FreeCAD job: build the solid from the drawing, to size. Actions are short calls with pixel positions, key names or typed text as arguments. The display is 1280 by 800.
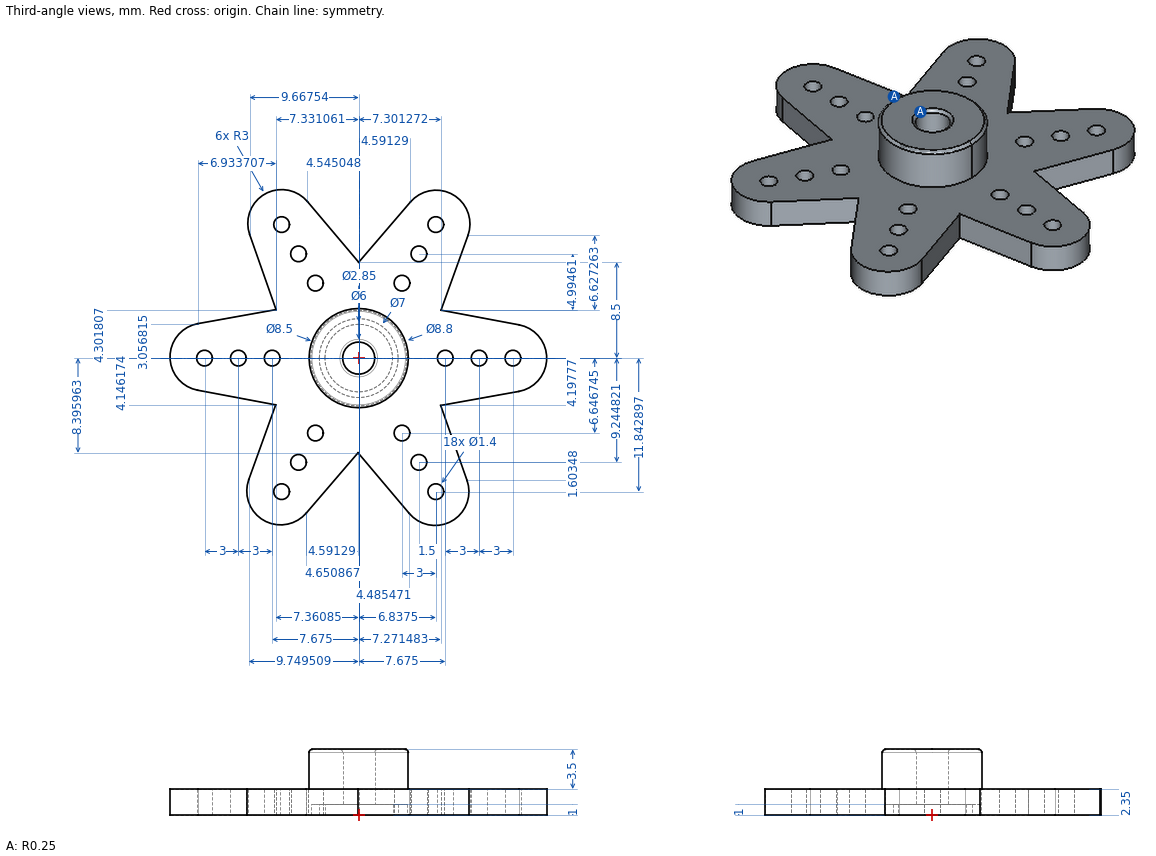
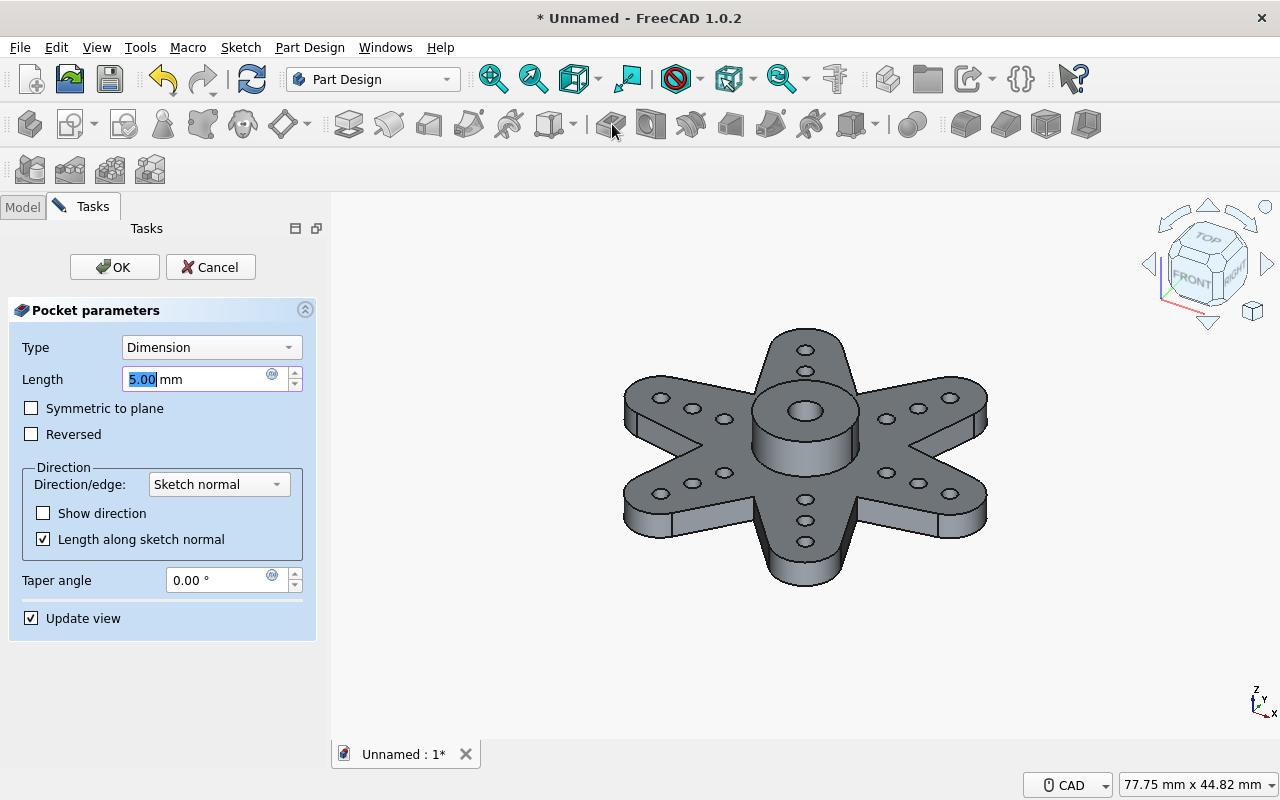
click(212, 348)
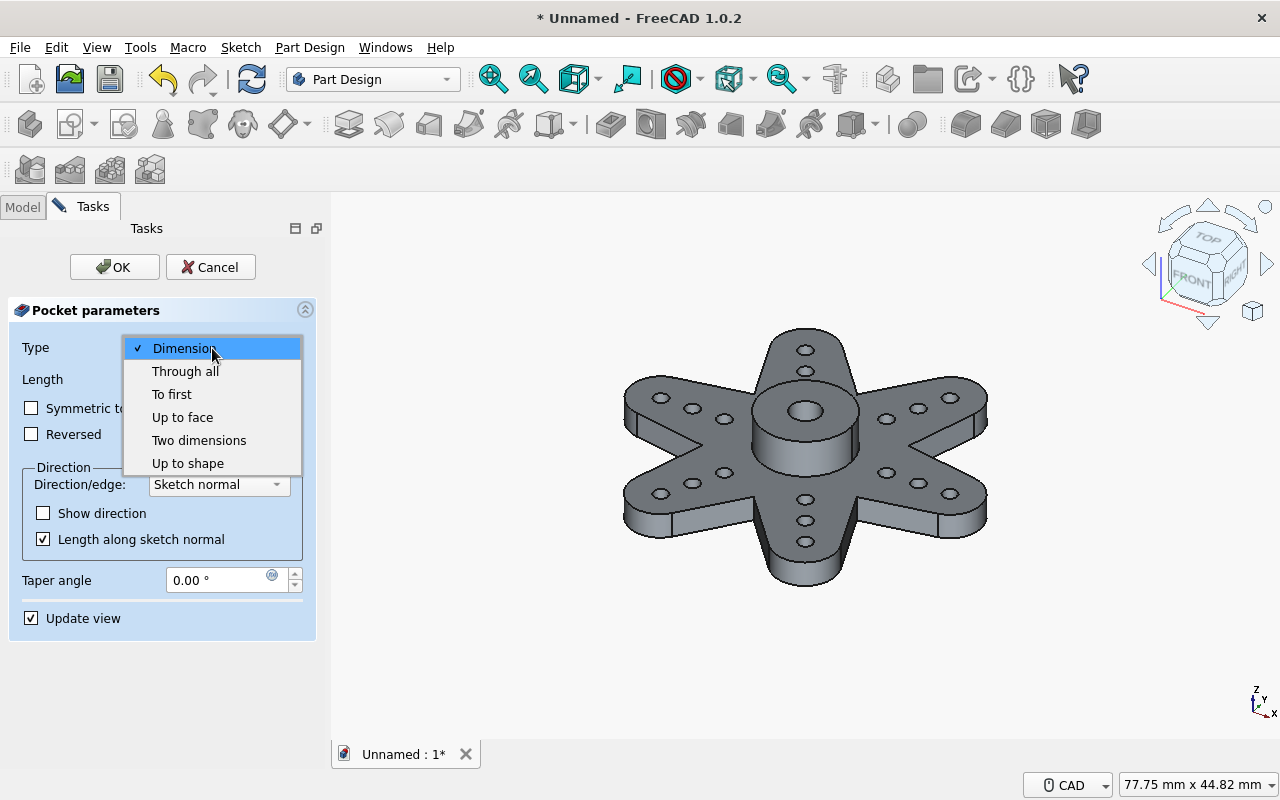
click(212, 372)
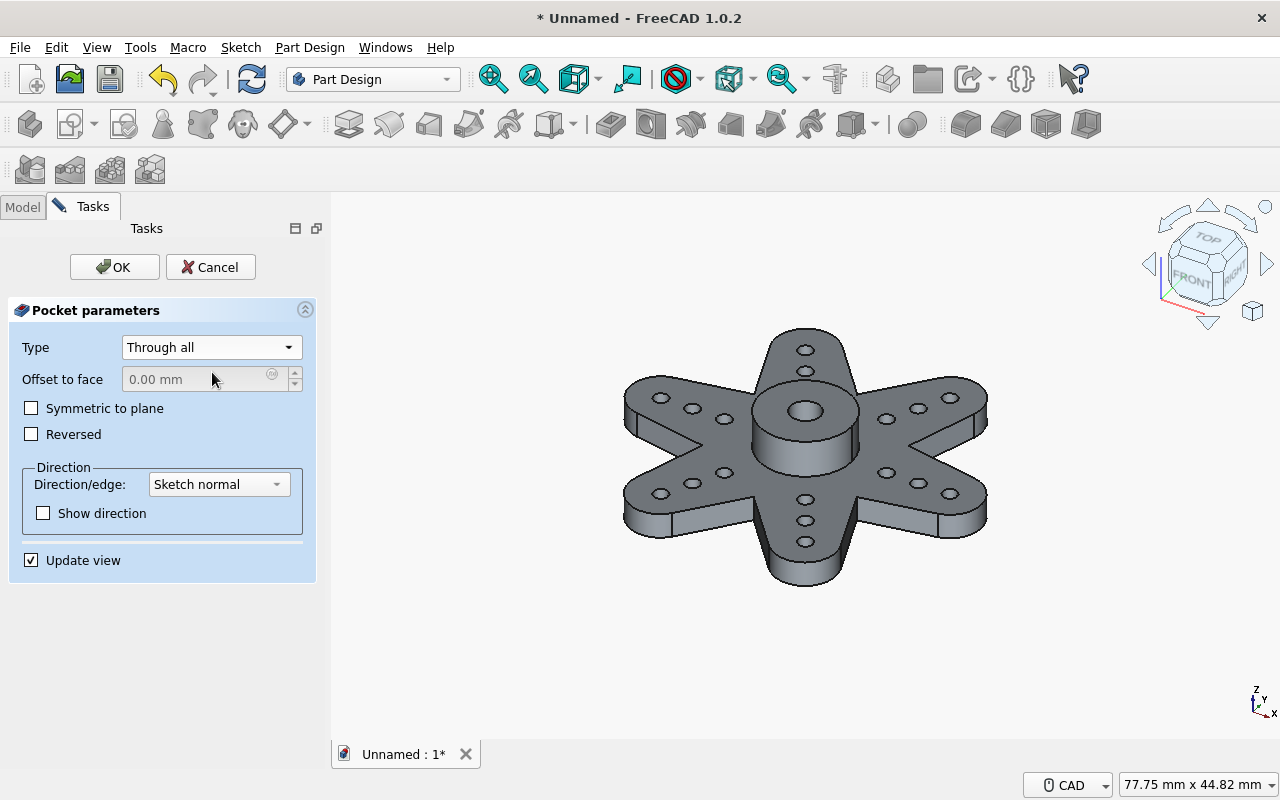
click(115, 267)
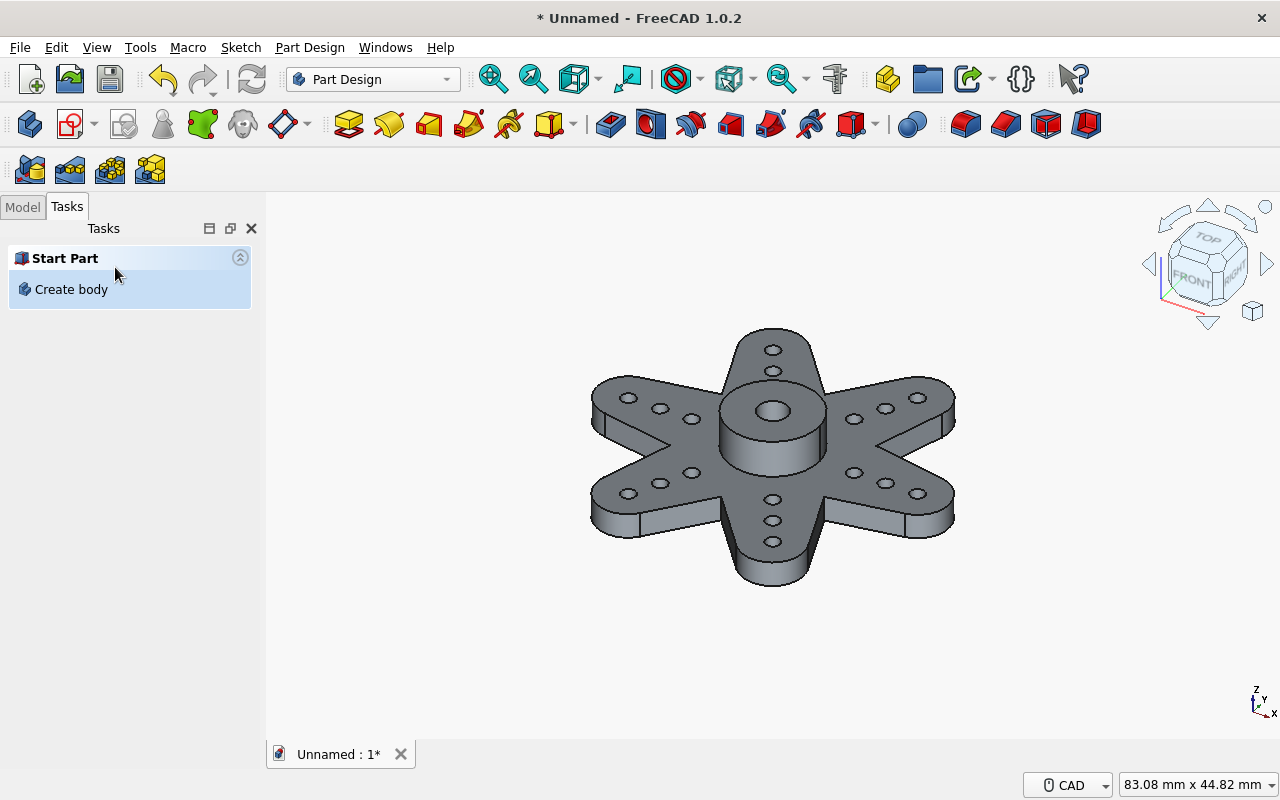
click(726, 395)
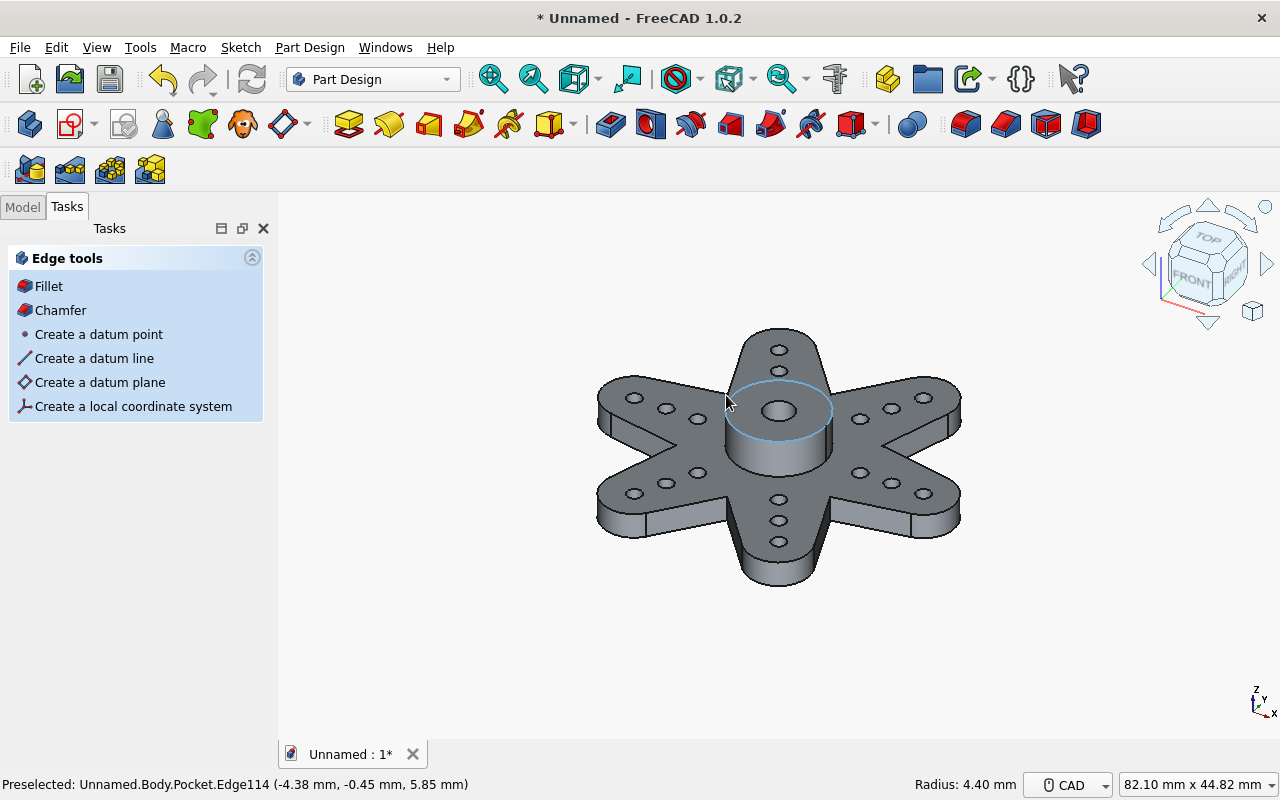
click(764, 405, ctrl)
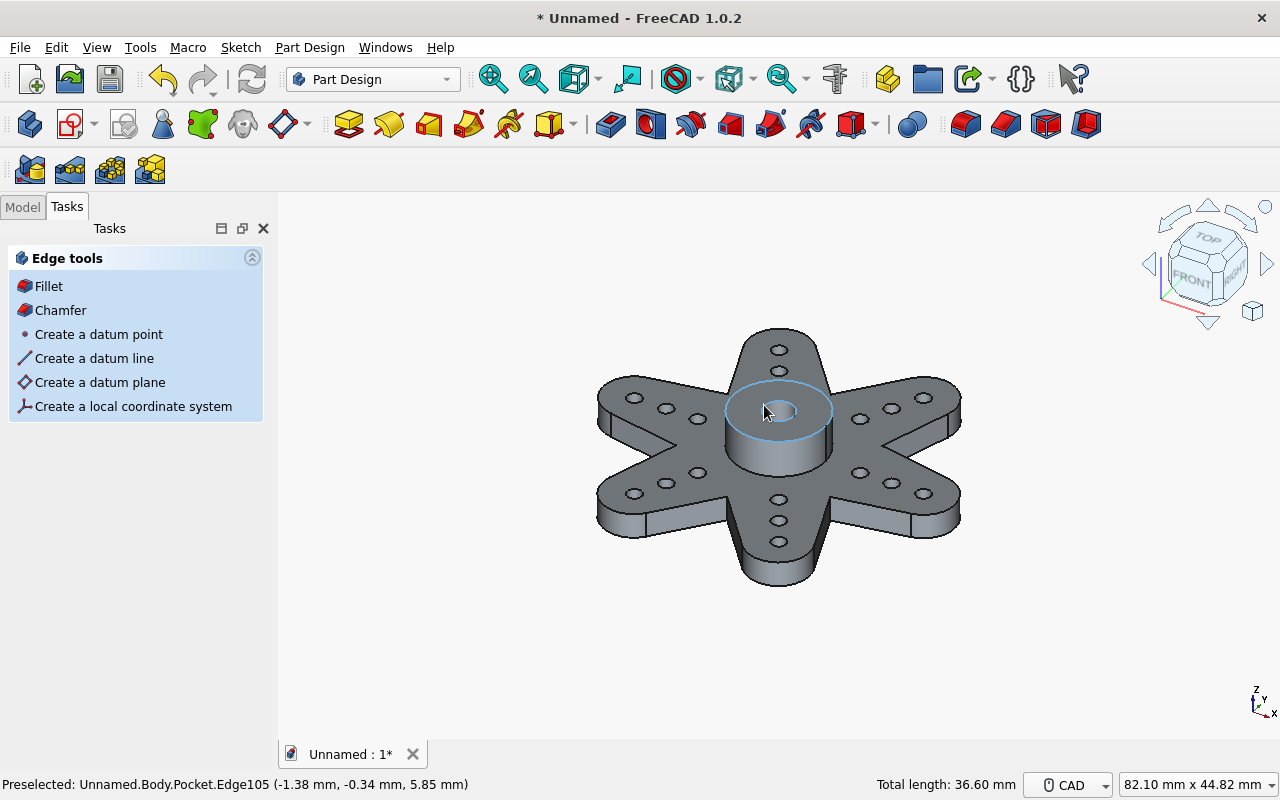
click(966, 124)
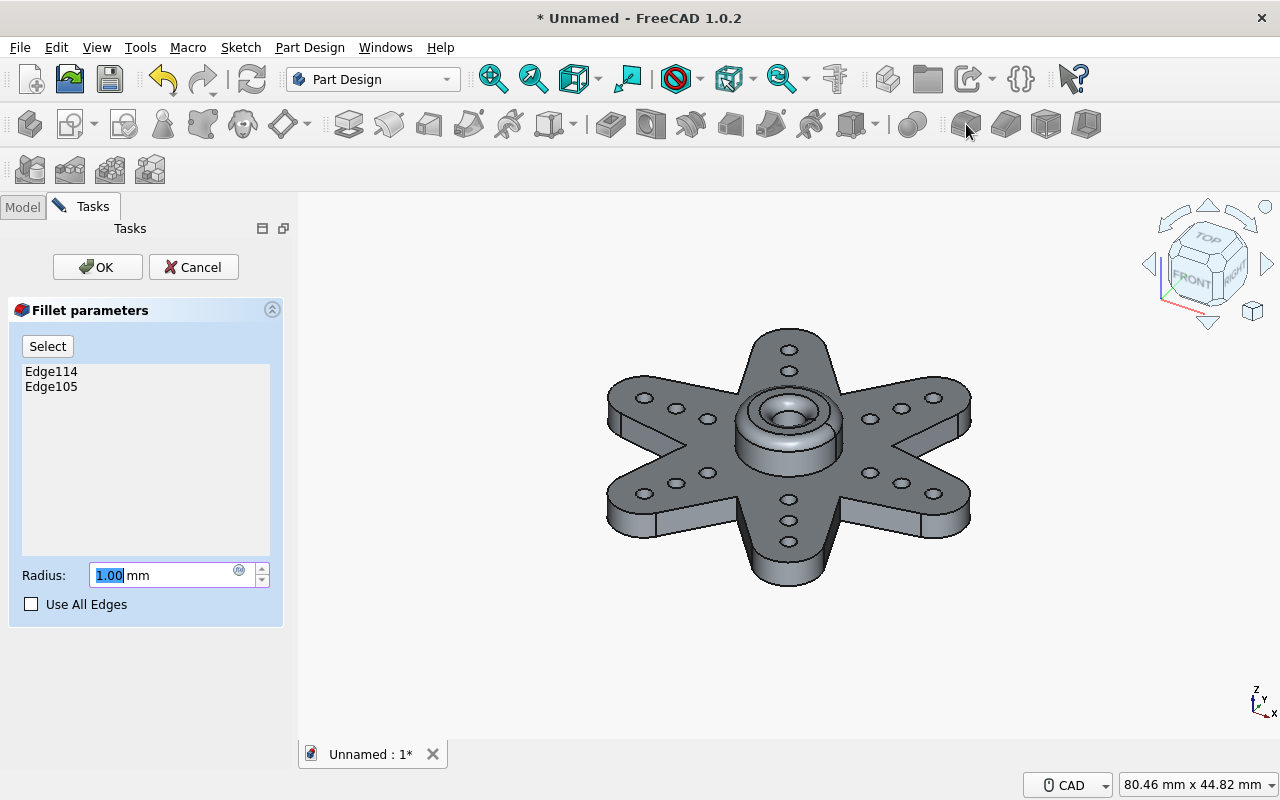
text(0.25)
key(Tab)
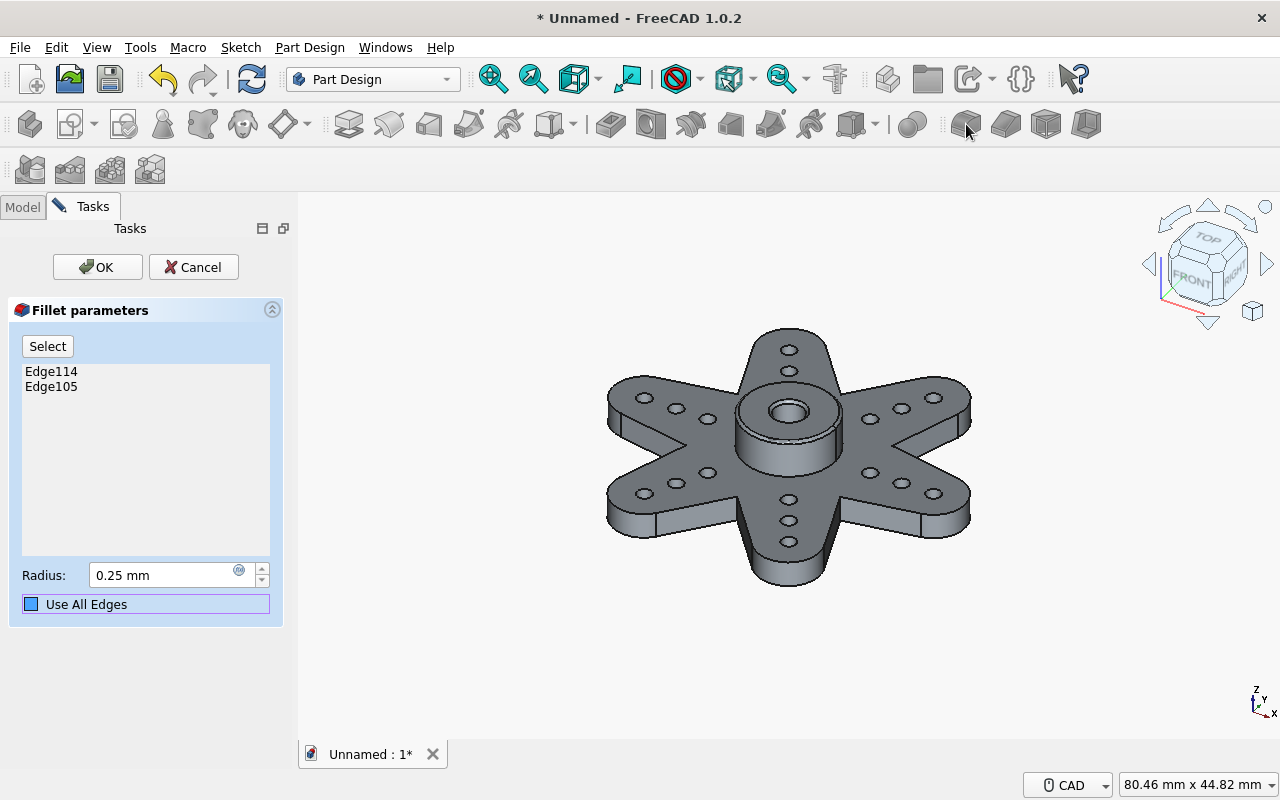
click(98, 267)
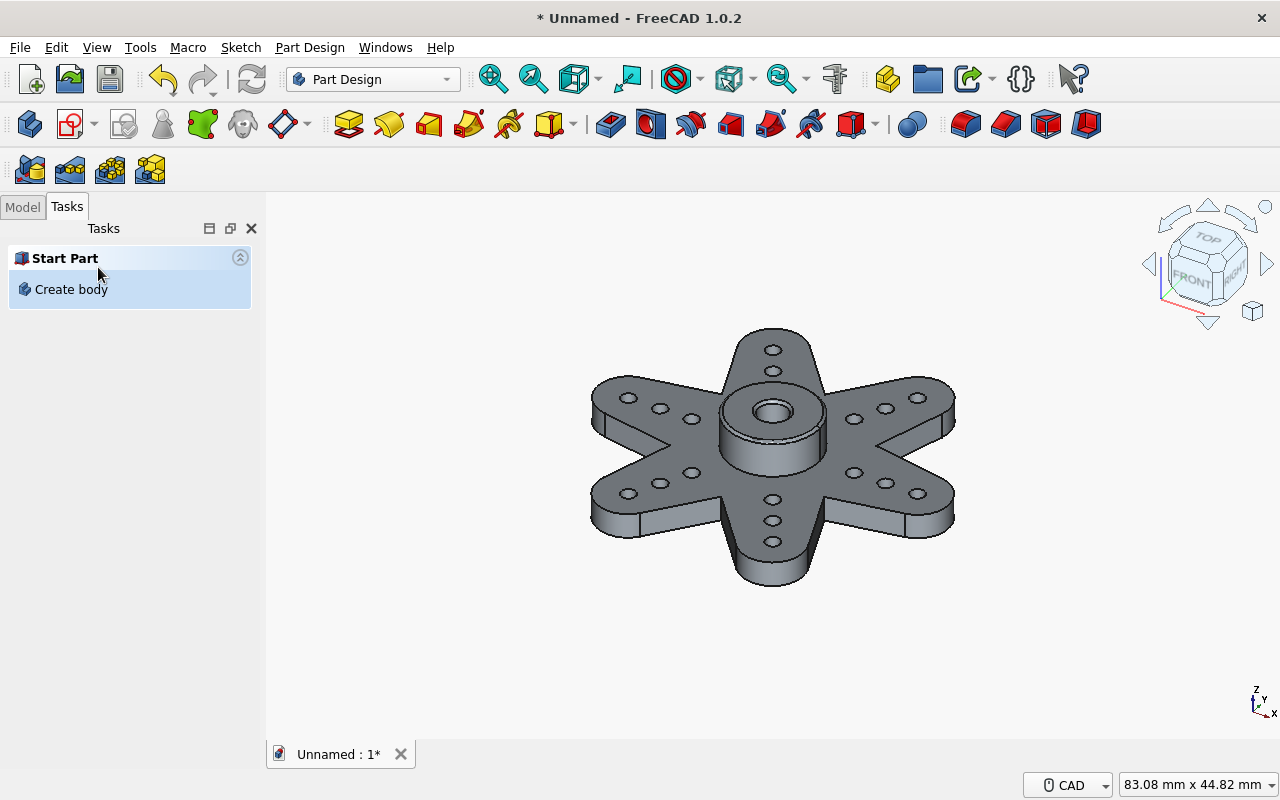
key(5)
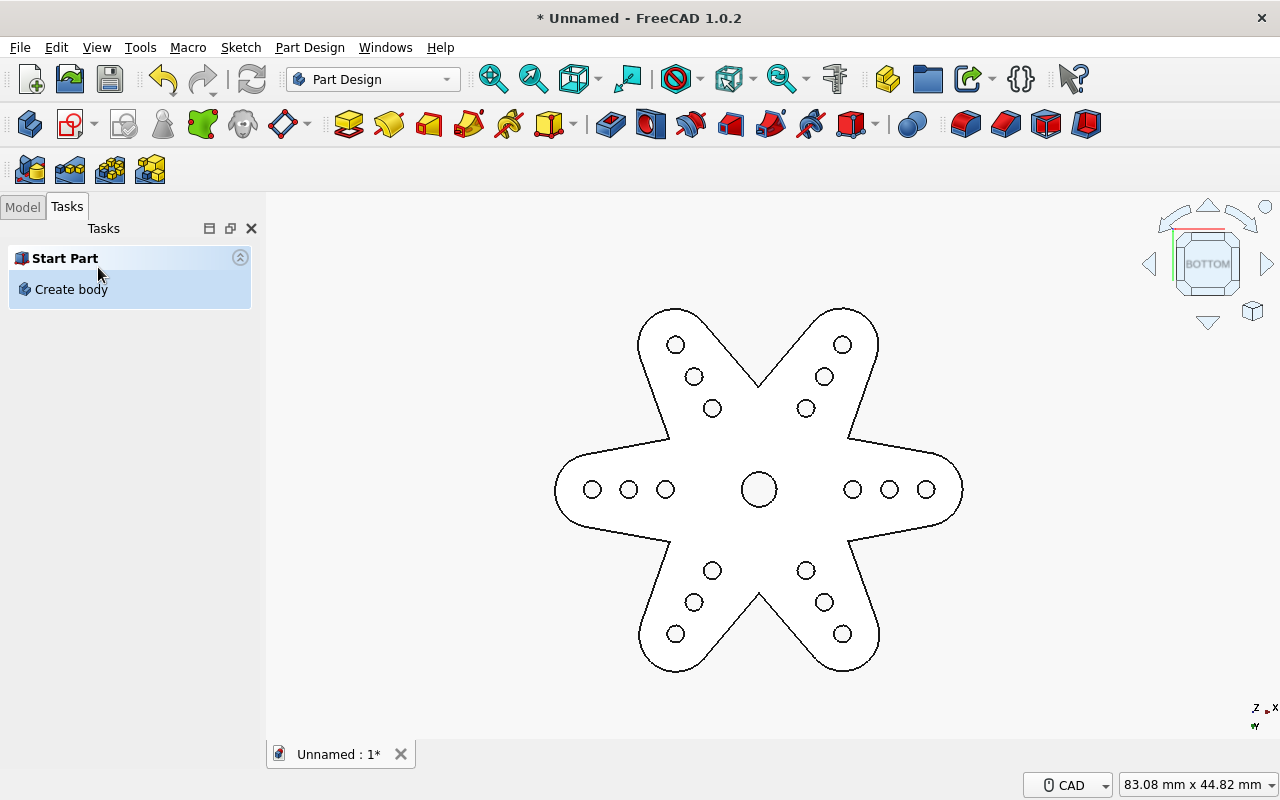
click(759, 541)